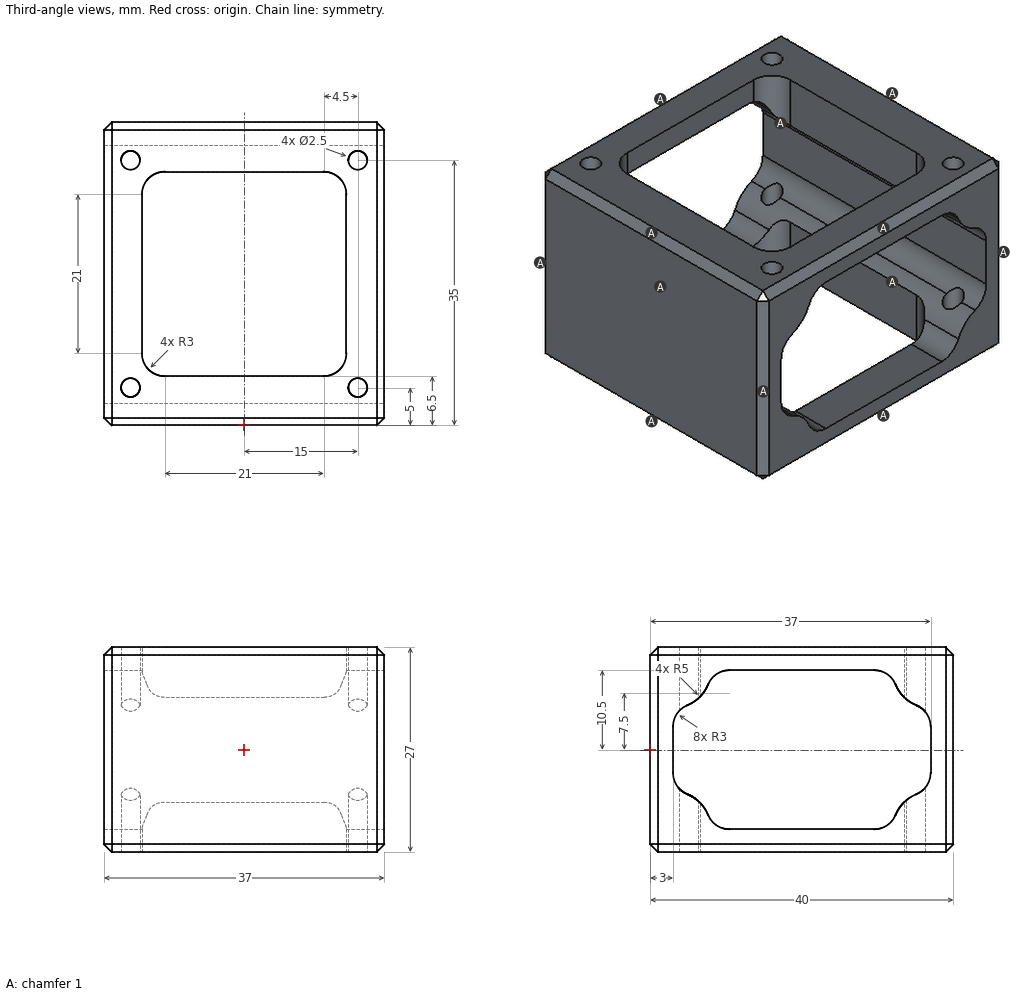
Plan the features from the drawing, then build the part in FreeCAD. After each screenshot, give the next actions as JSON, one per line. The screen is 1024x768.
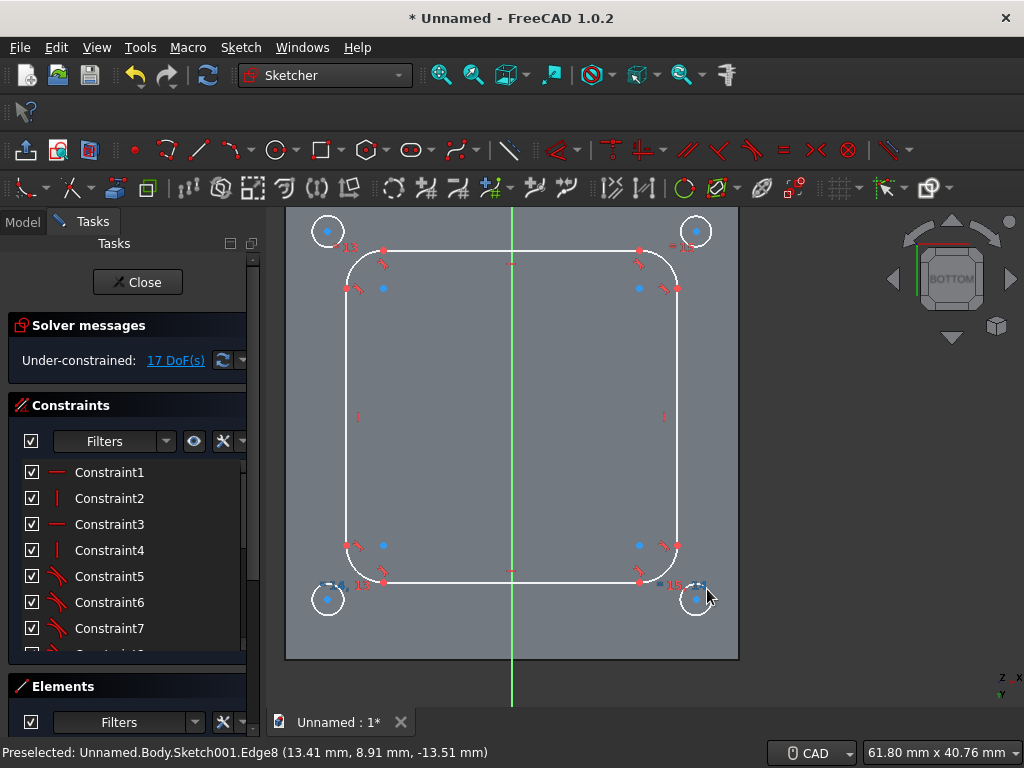
{"action": "left_click", "coordinate": [707, 589]}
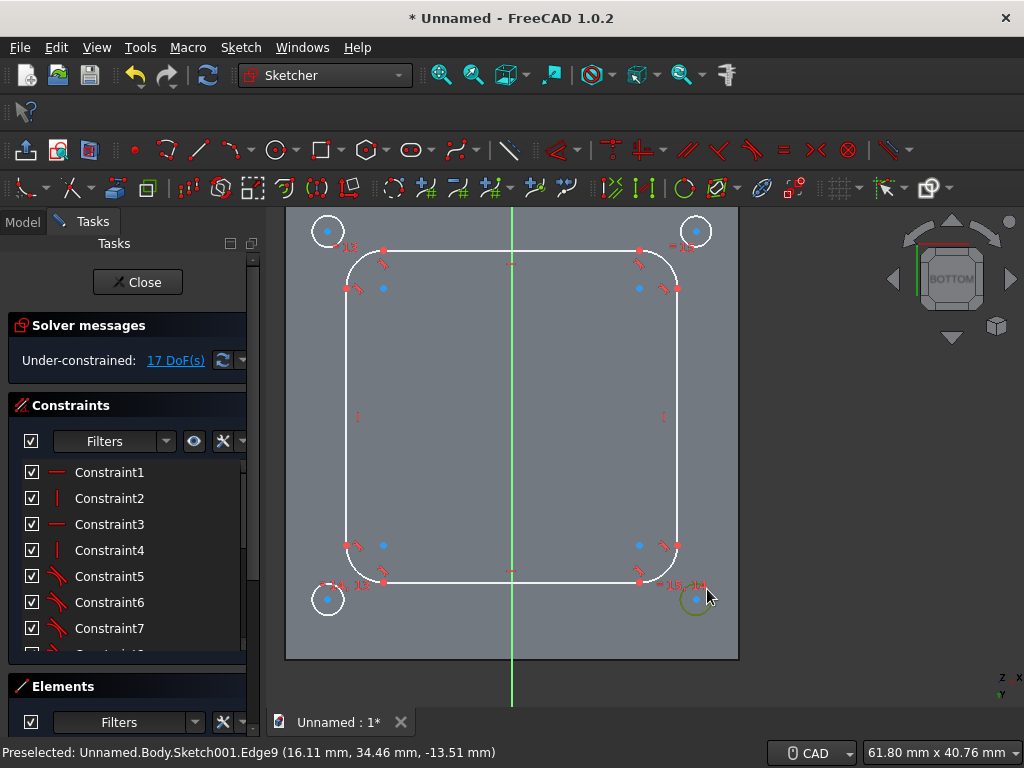
{"action": "left_click", "coordinate": [317, 589]}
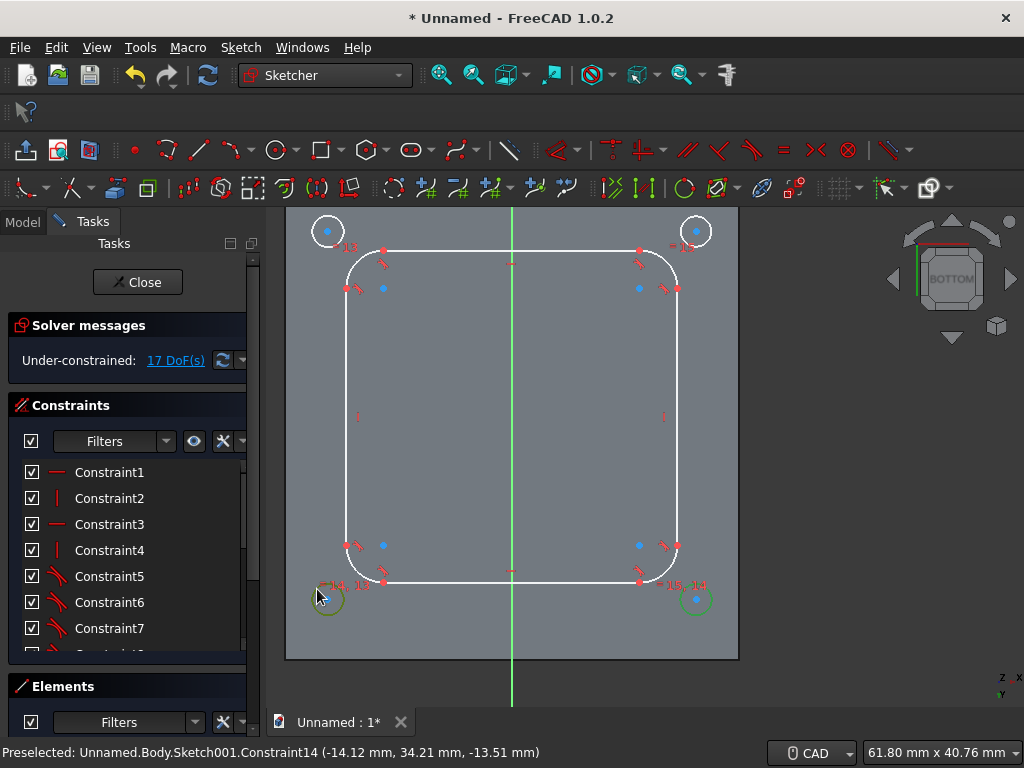
{"action": "left_click", "coordinate": [707, 242]}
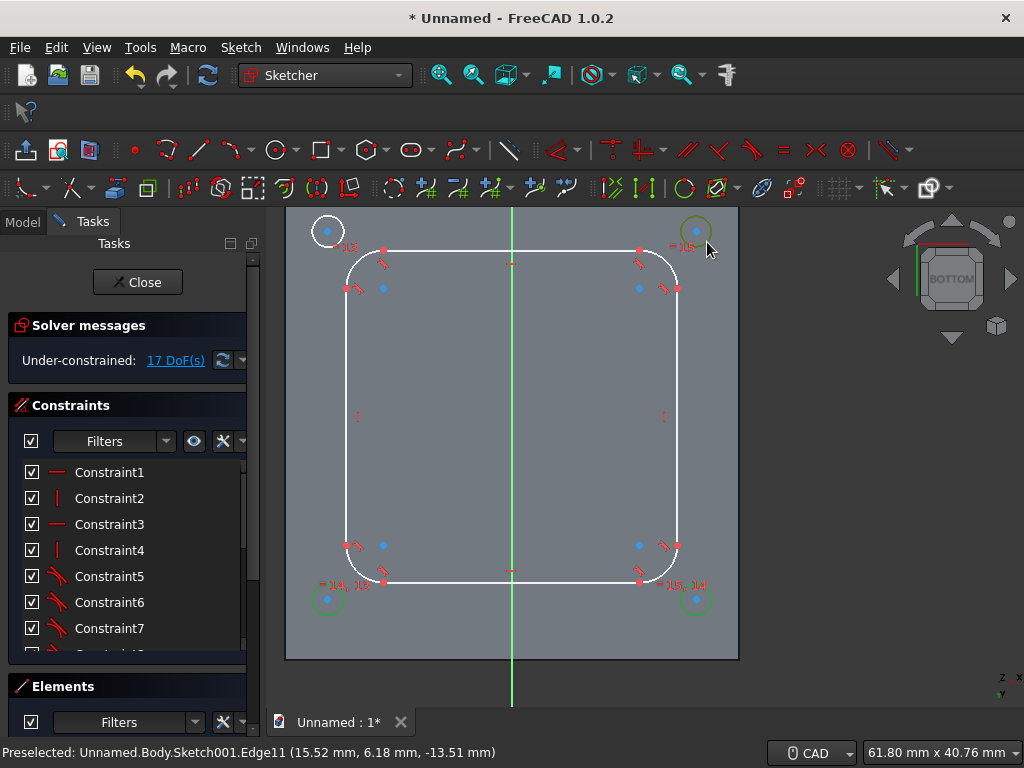
{"action": "left_click", "coordinate": [317, 243]}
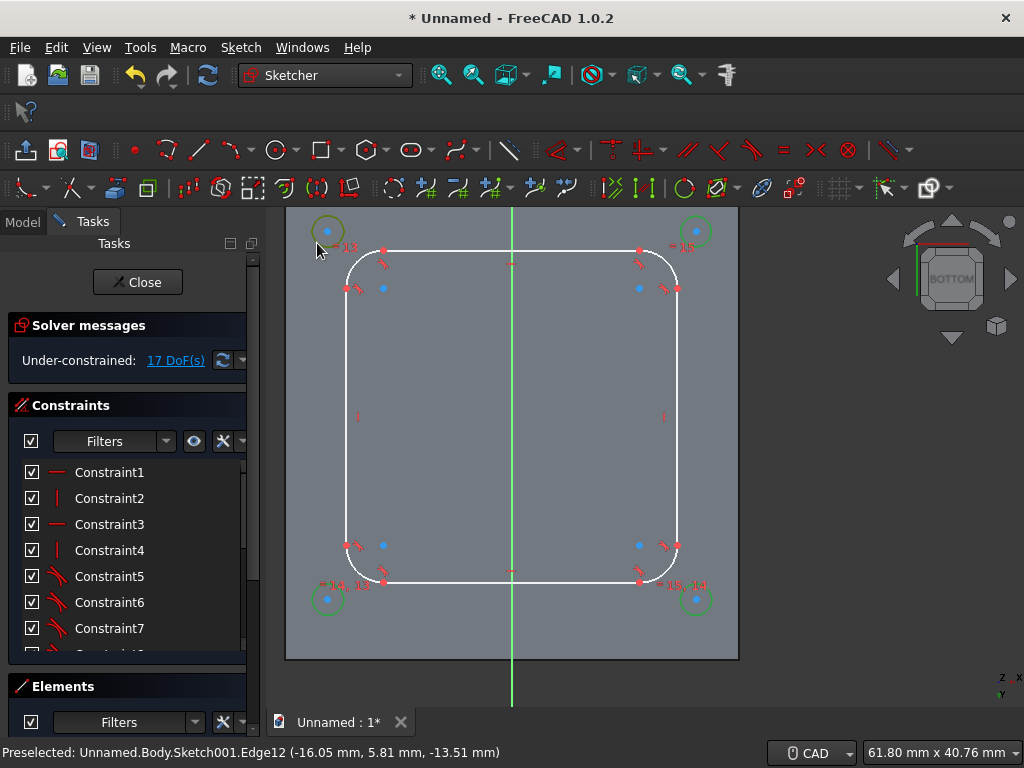
{"action": "key", "text": "e"}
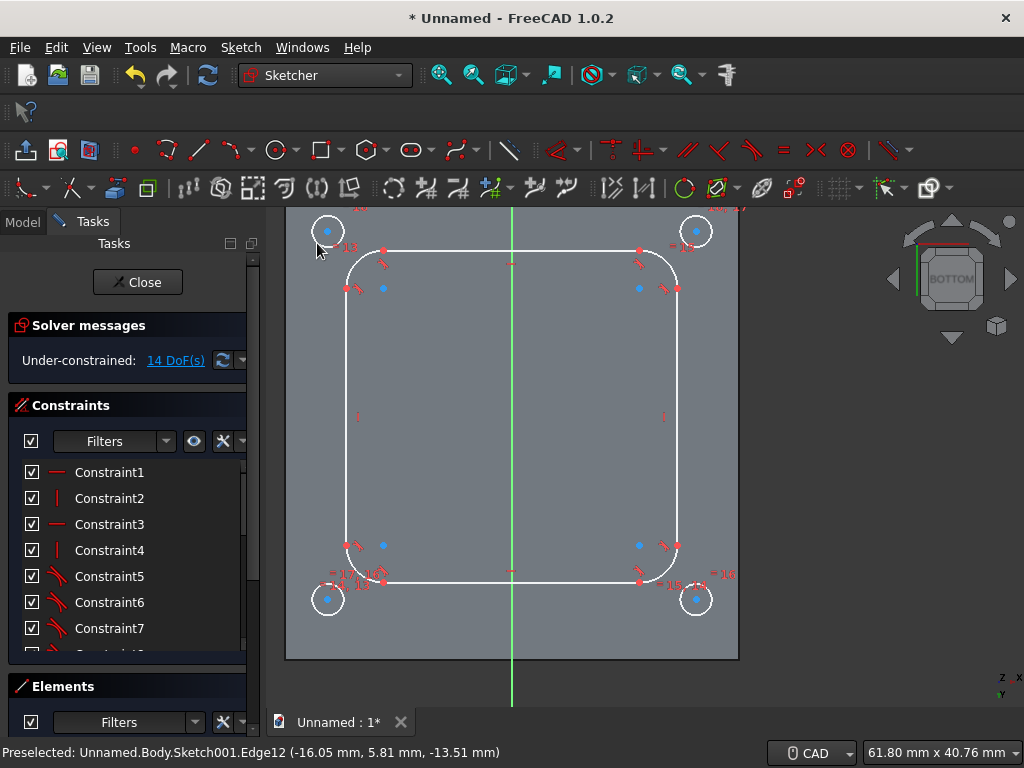
{"action": "left_click", "coordinate": [696, 600]}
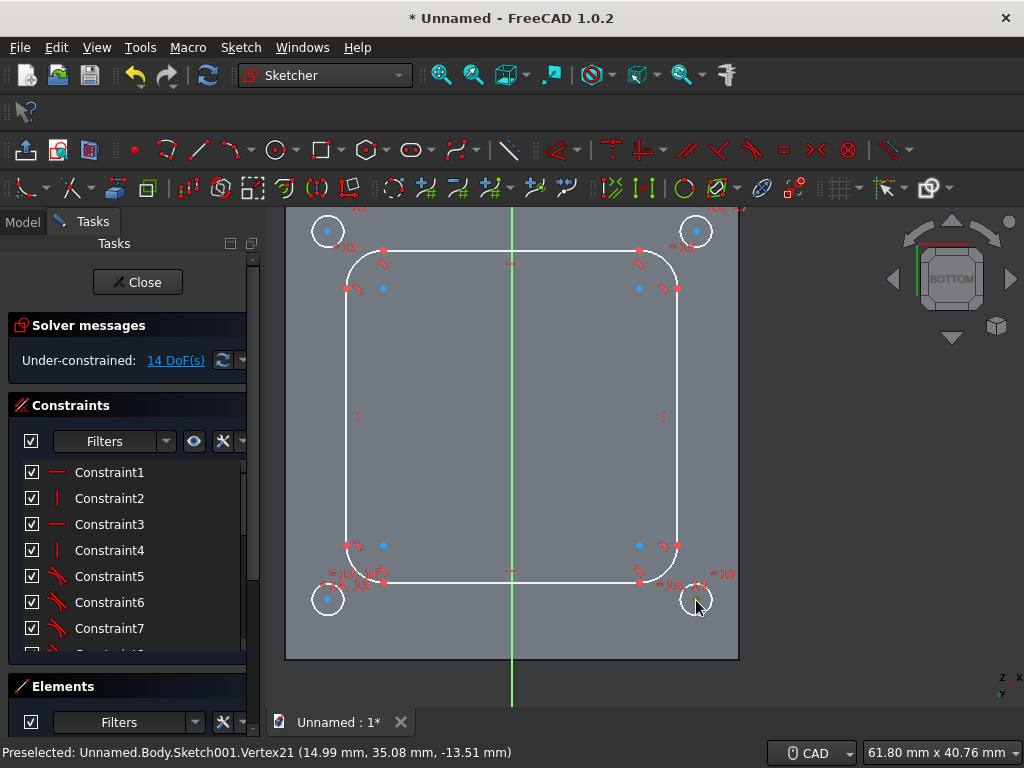
{"action": "left_click", "coordinate": [328, 600]}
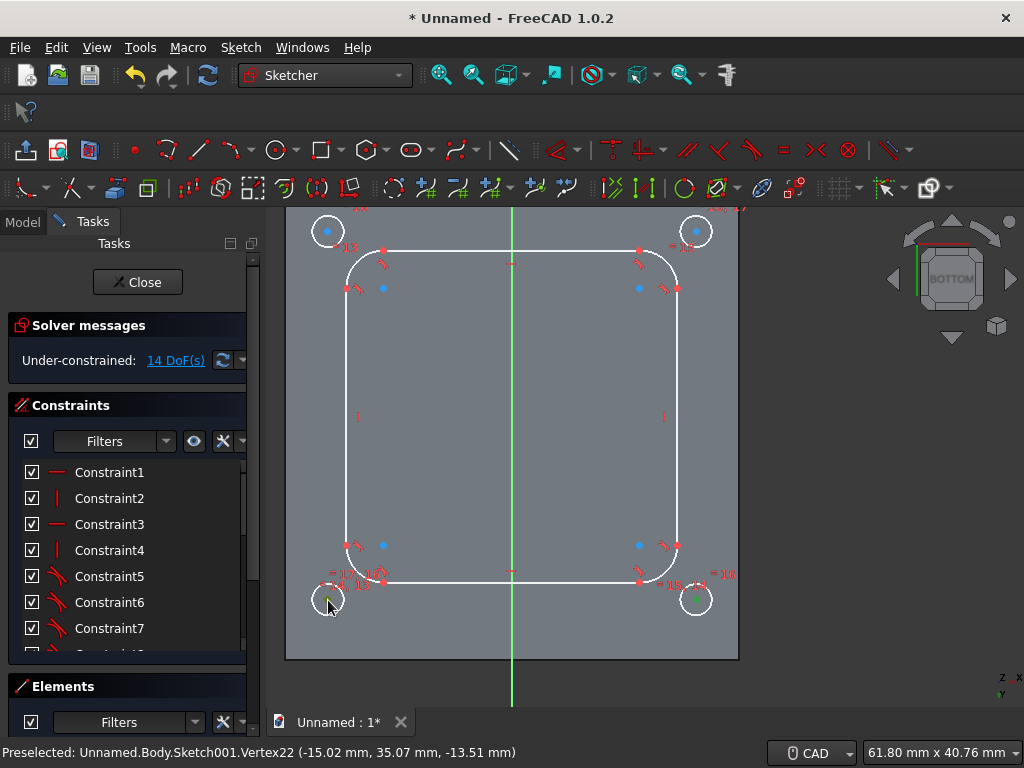
{"action": "left_click", "coordinate": [512, 647]}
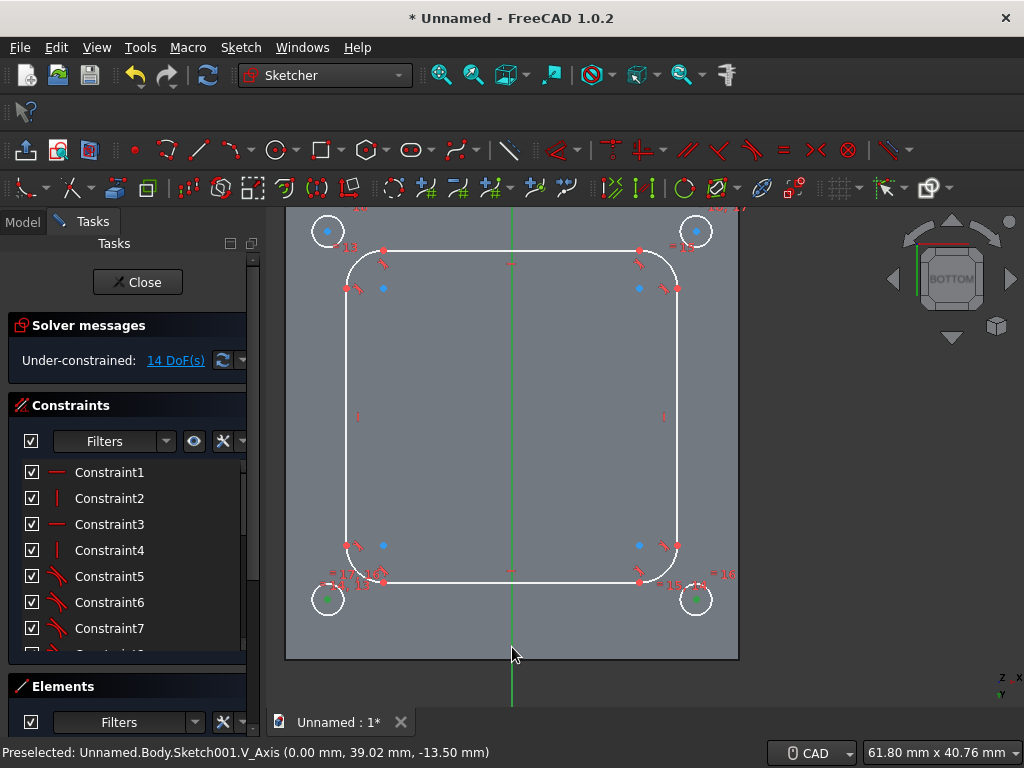
{"action": "key", "text": "s"}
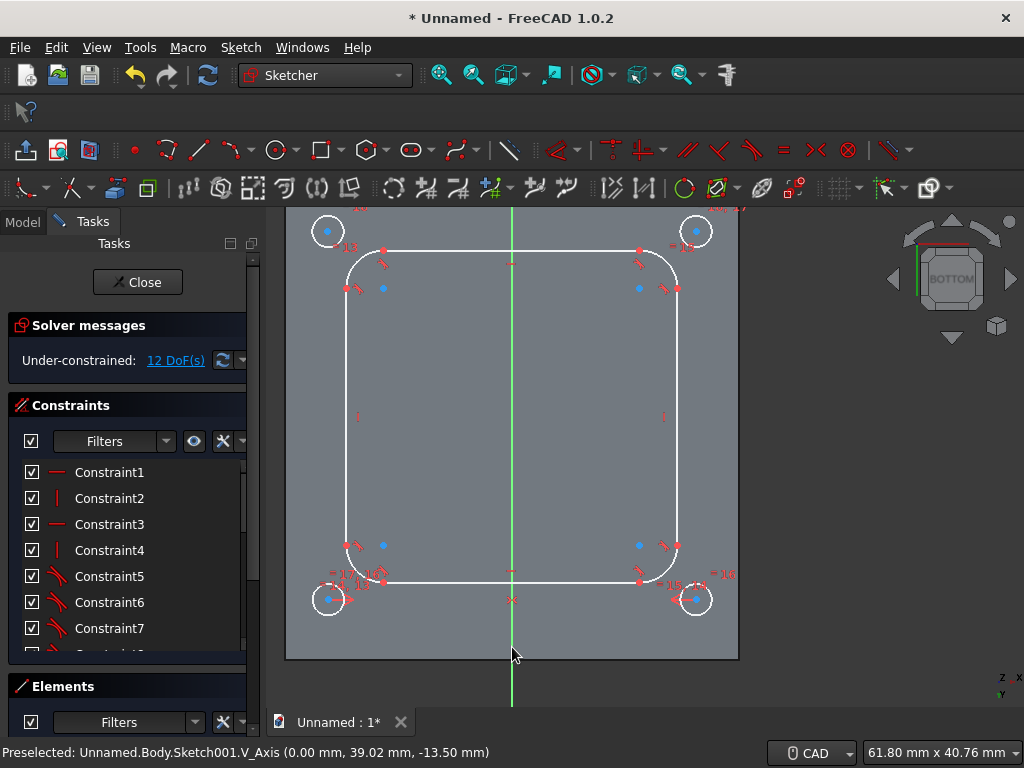
{"action": "scroll", "coordinate": [707, 590], "scroll_direction": "down", "scroll_amount": 2}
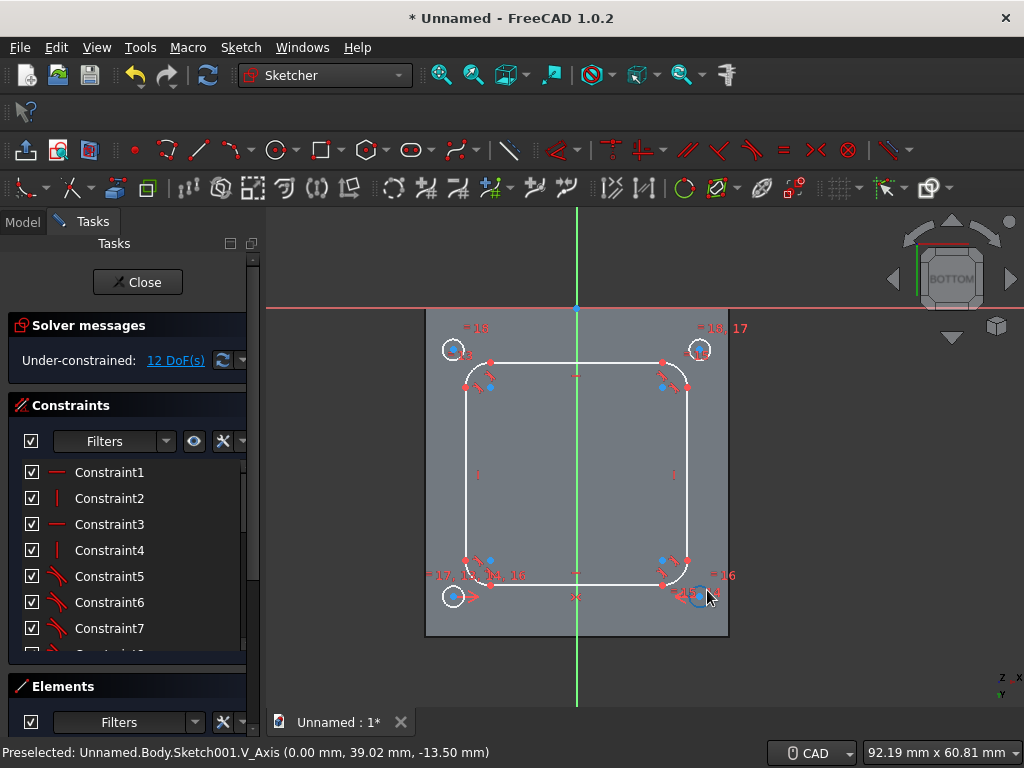
{"action": "scroll", "coordinate": [700, 350], "scroll_direction": "up", "scroll_amount": 4}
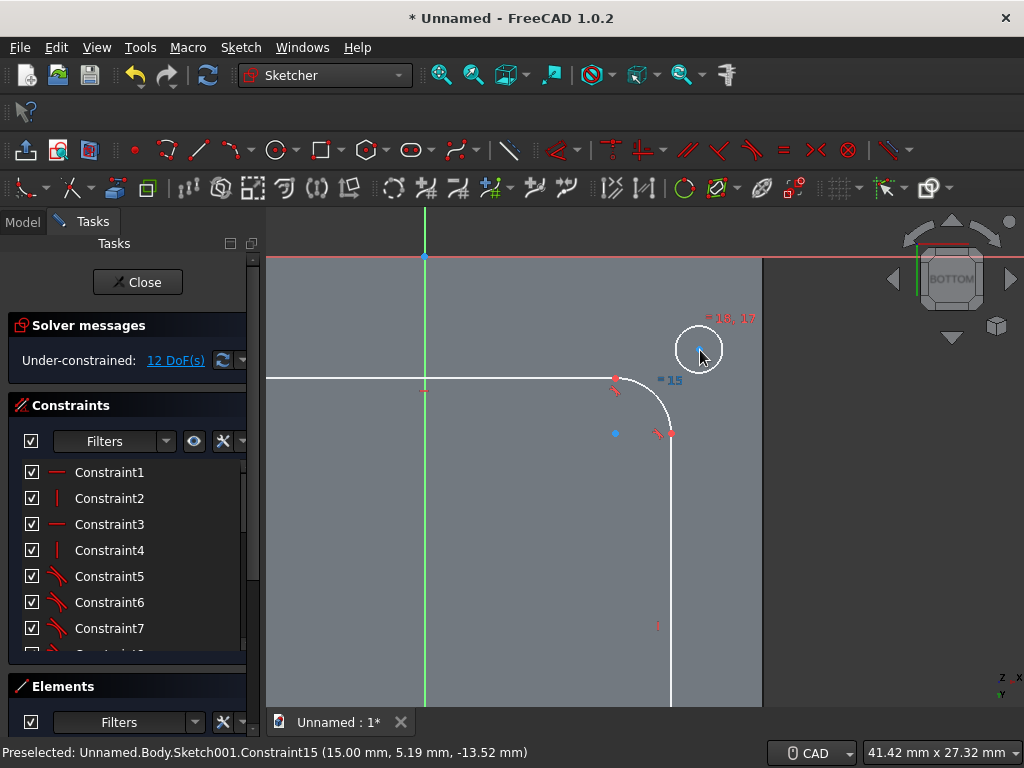
{"action": "left_click", "coordinate": [699, 350]}